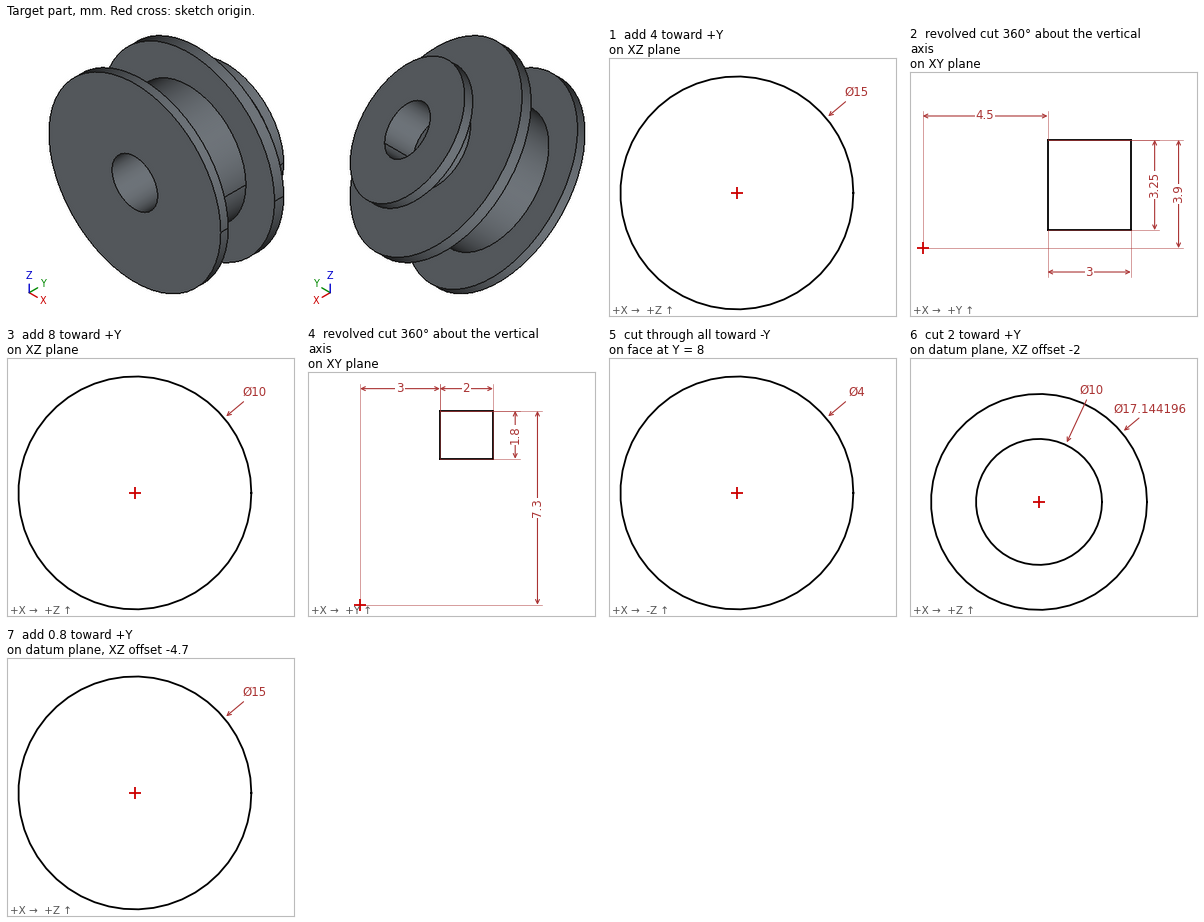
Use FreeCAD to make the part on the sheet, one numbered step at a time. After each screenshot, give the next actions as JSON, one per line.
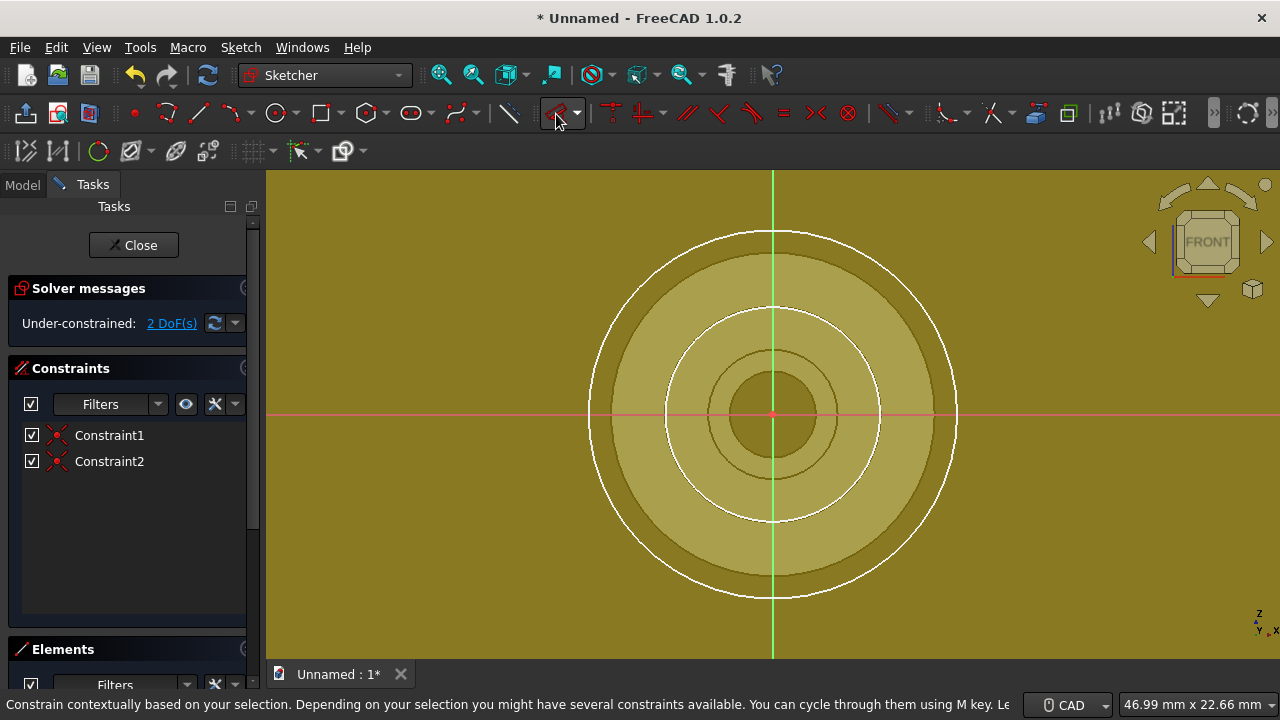
{"action": "left_click", "coordinate": [903, 284]}
{"action": "left_click", "coordinate": [926, 261]}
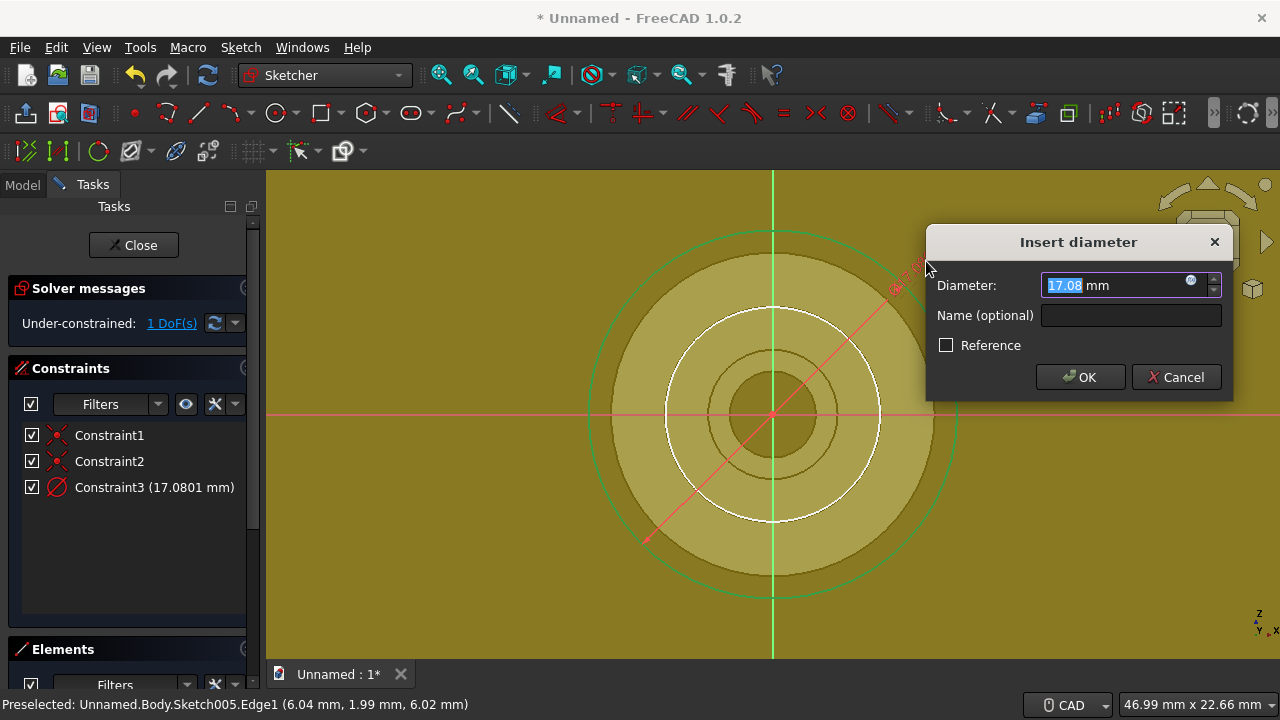
{"action": "type", "text": "17.144196"}
{"action": "key", "text": "Return"}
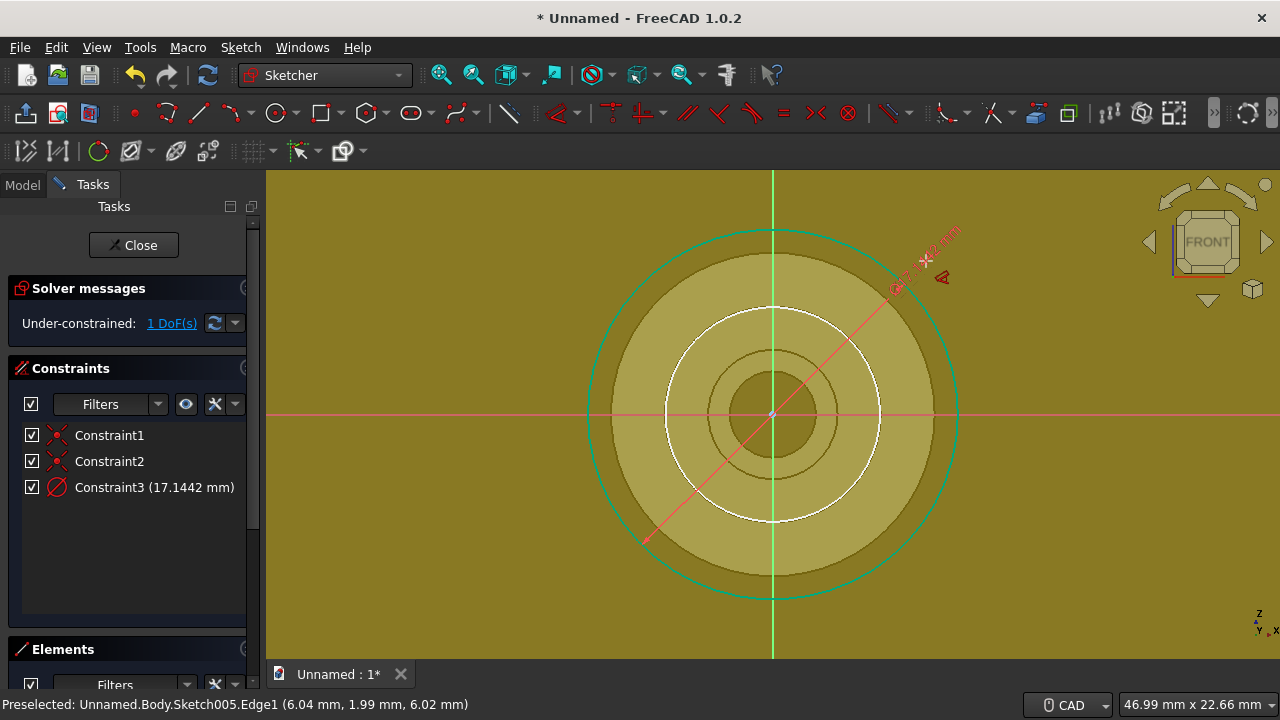
{"action": "left_click", "coordinate": [848, 338]}
{"action": "left_click", "coordinate": [870, 315]}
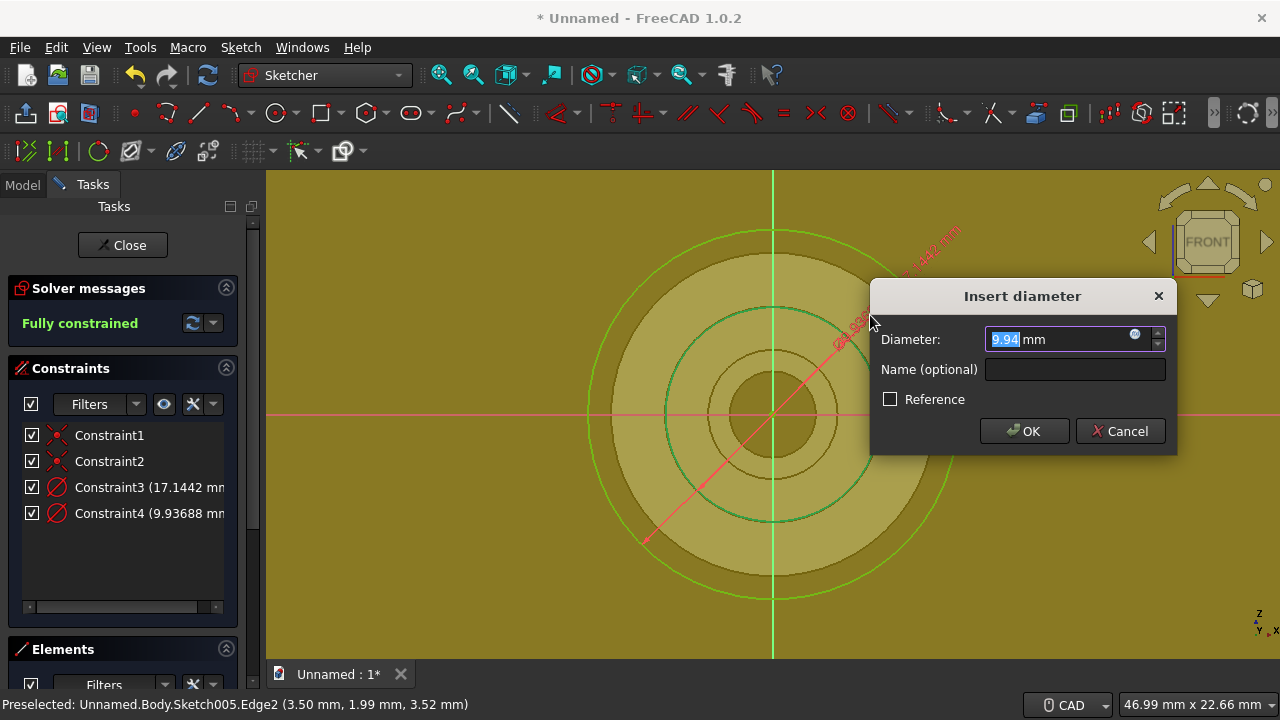
{"action": "type", "text": "10"}
{"action": "key", "text": "Return"}
{"action": "key", "text": "Escape"}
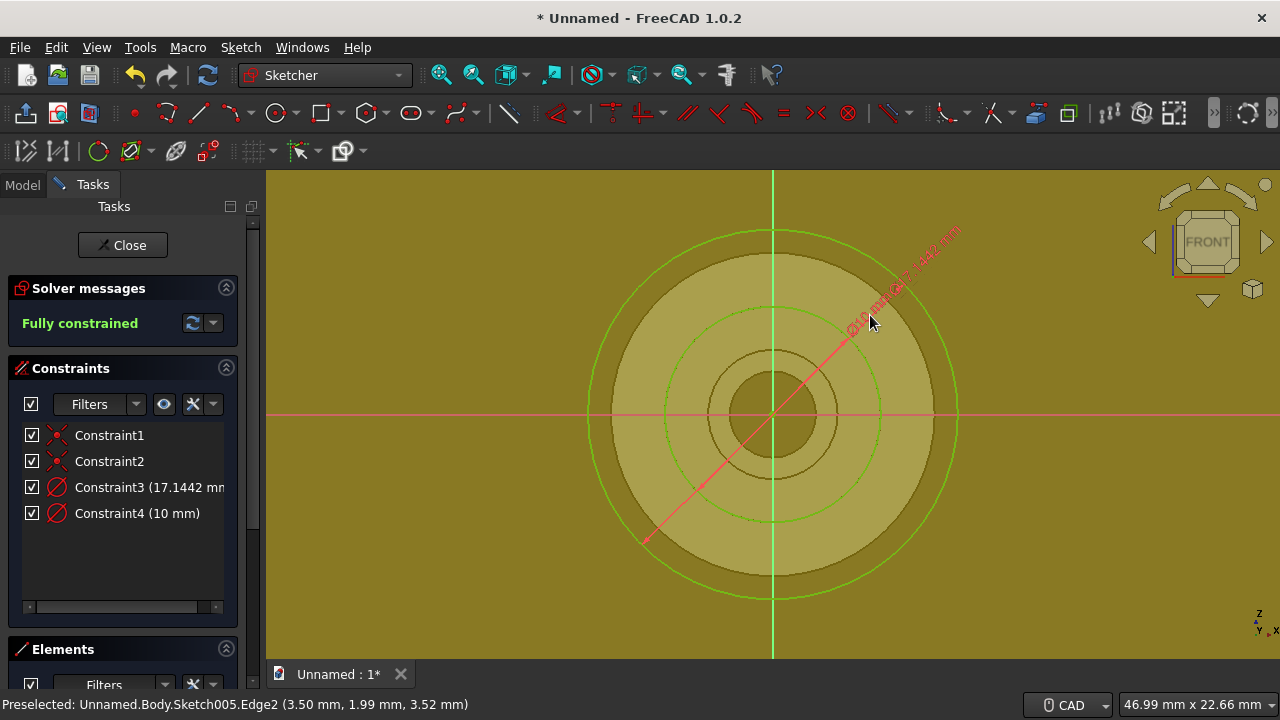
{"action": "left_click", "coordinate": [123, 245]}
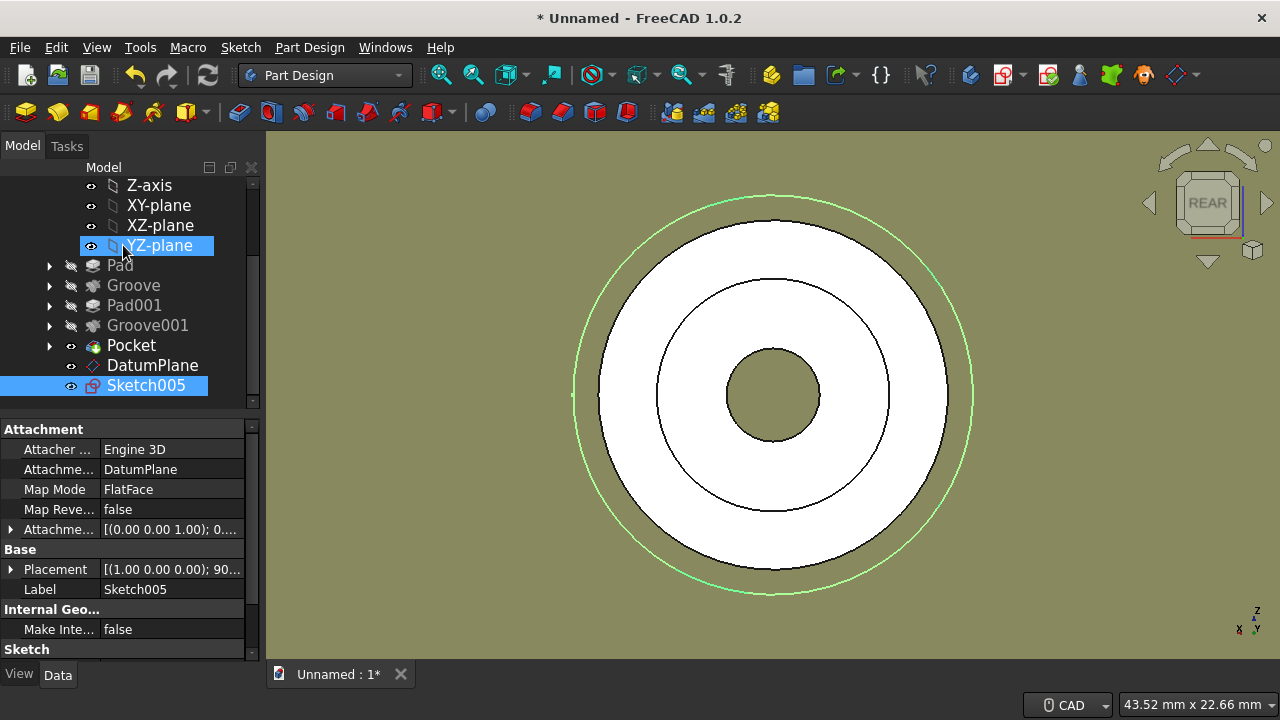
{"action": "left_click", "coordinate": [240, 112]}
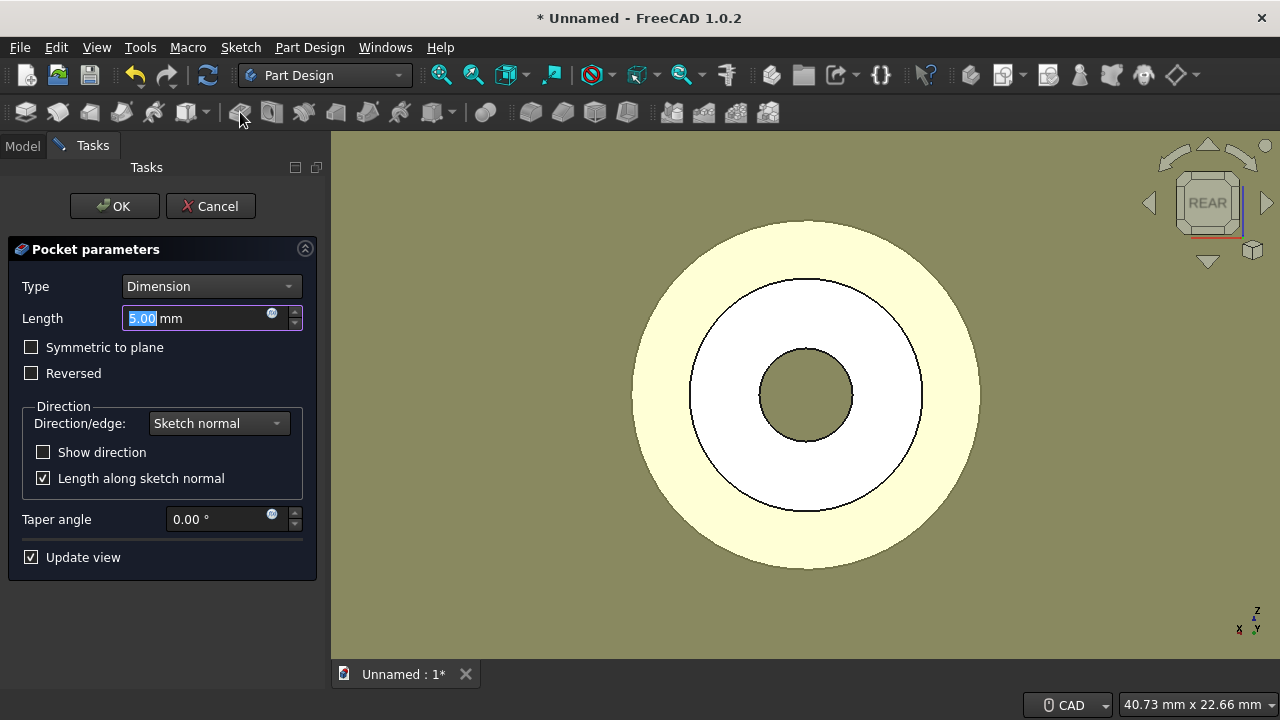
{"action": "type", "text": "2"}
{"action": "key", "text": "Tab"}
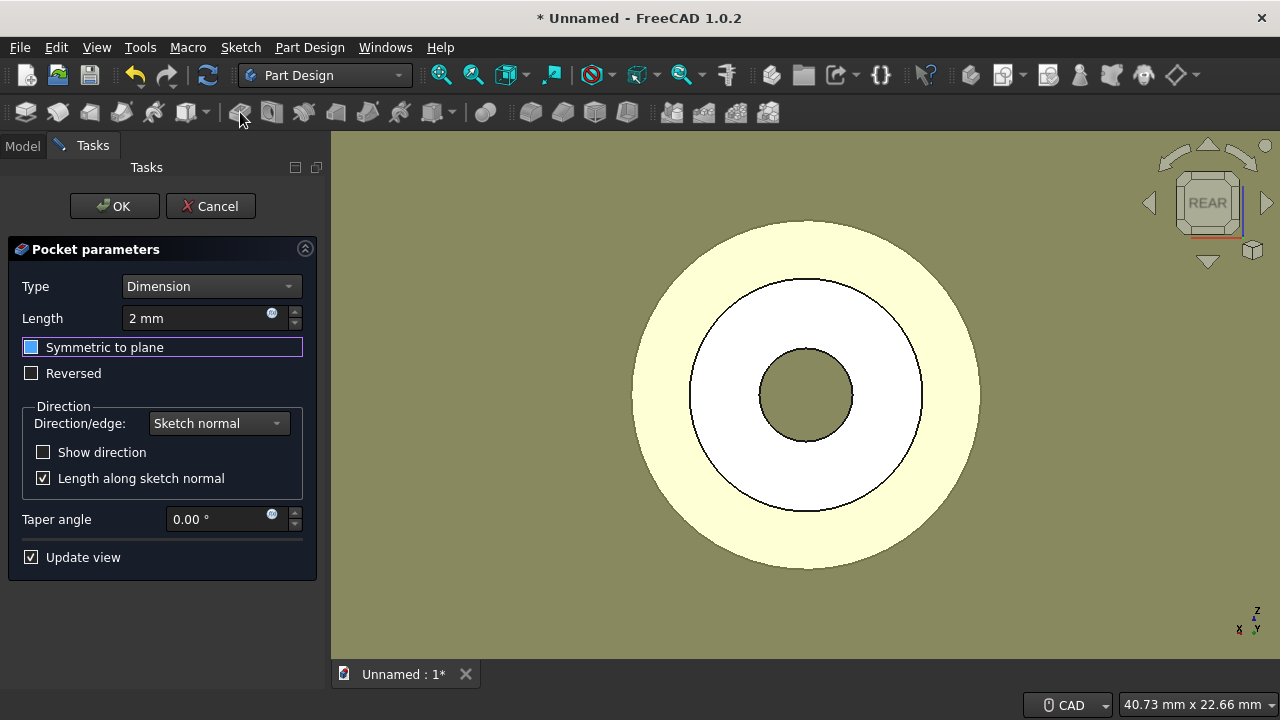
{"action": "left_click", "coordinate": [115, 206]}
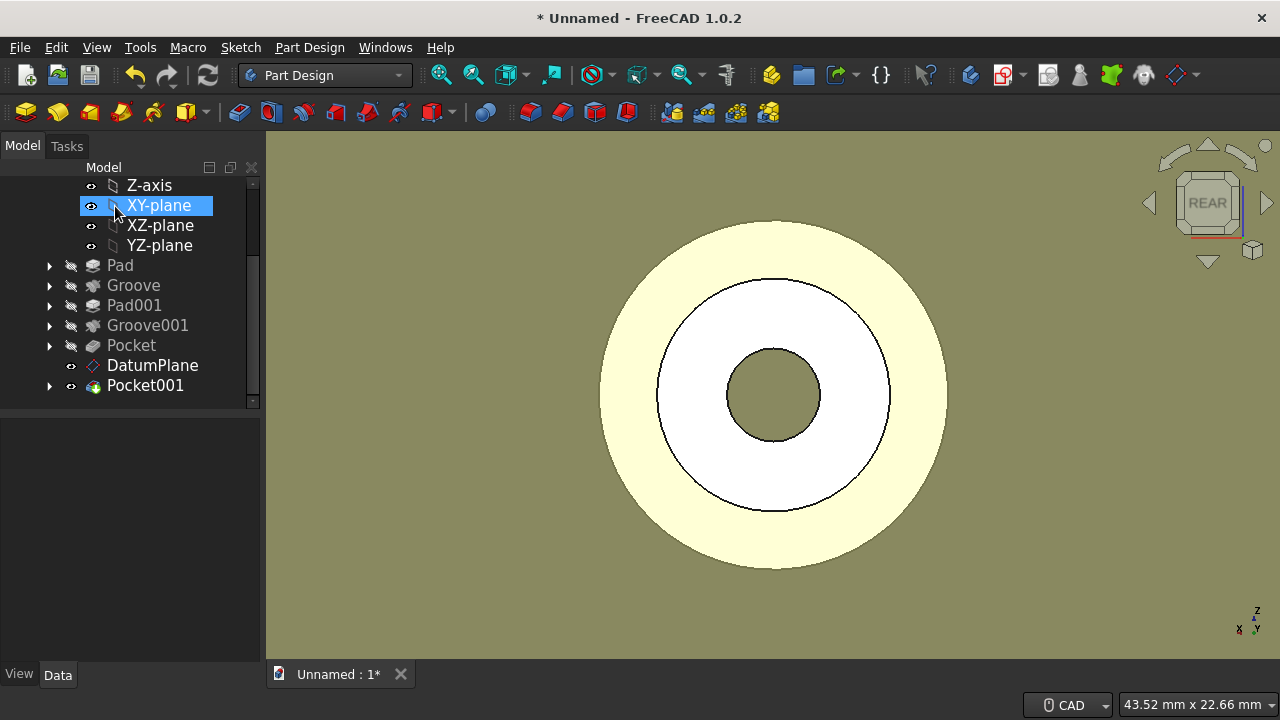
{"action": "left_click", "coordinate": [116, 366]}
{"action": "key", "text": "space"}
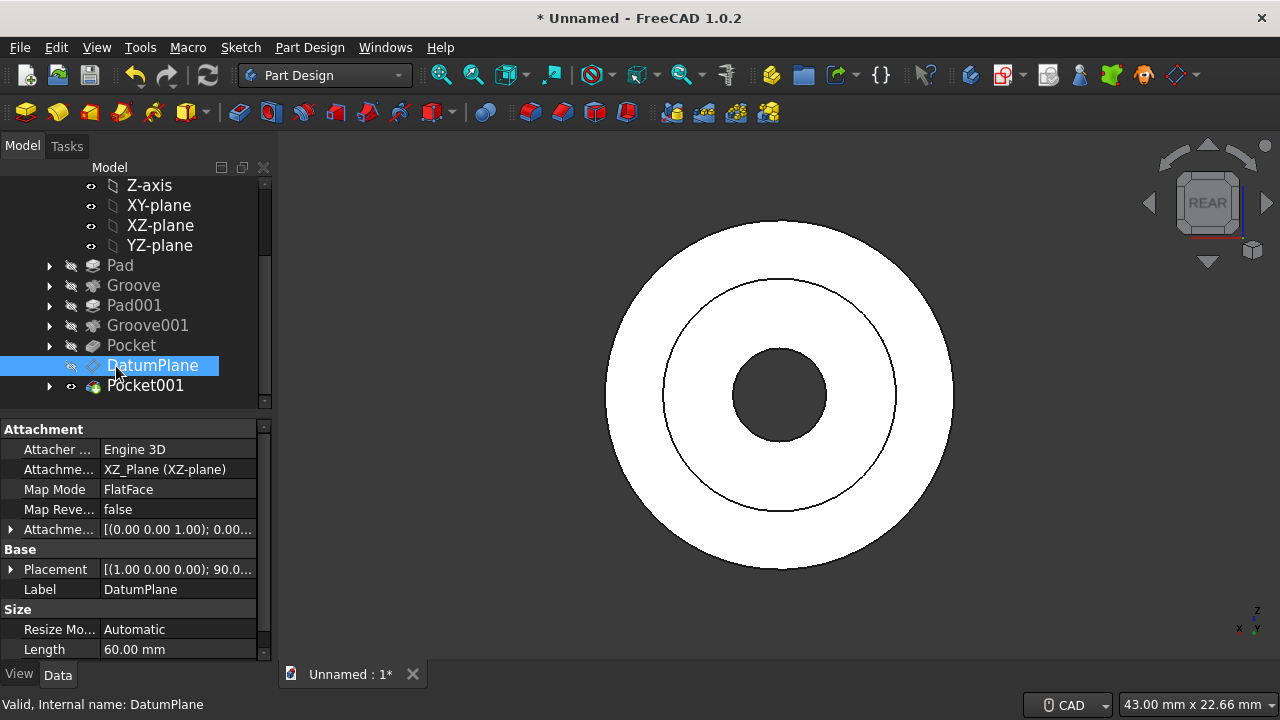
{"action": "scroll", "coordinate": [160, 281], "scroll_direction": "down", "scroll_amount": 3}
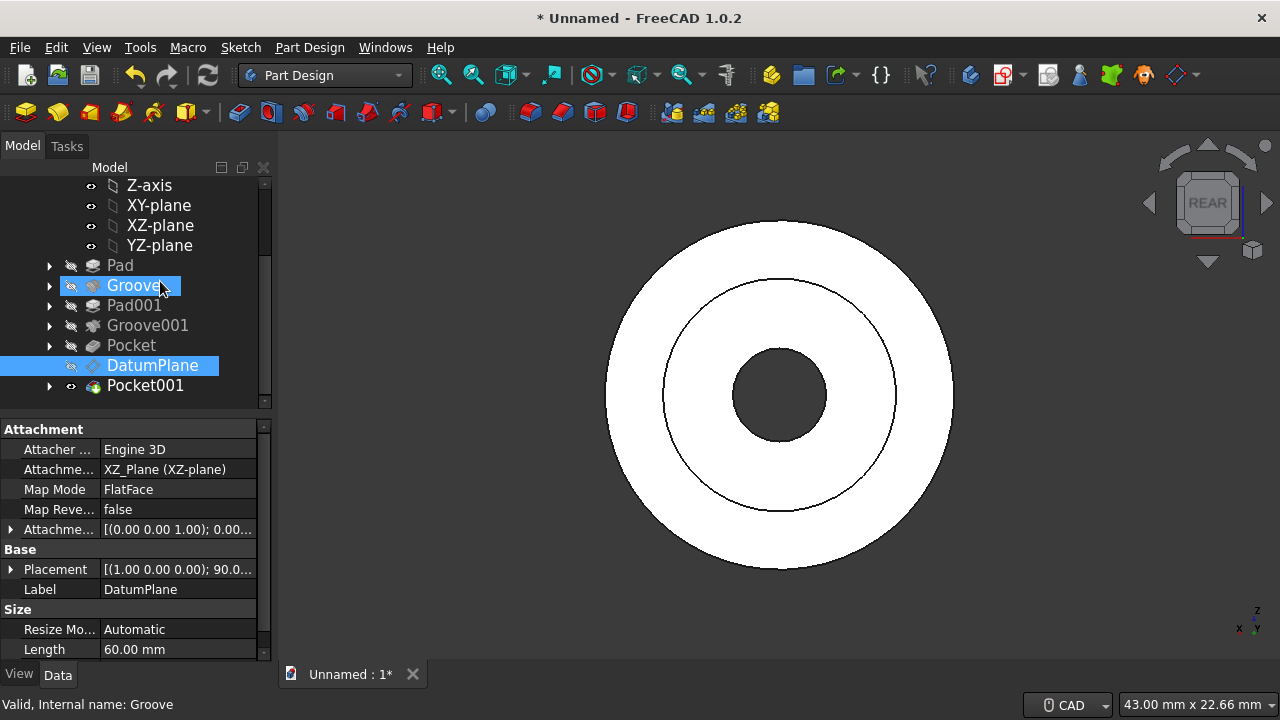
{"action": "scroll", "coordinate": [160, 281], "scroll_direction": "up", "scroll_amount": 15}